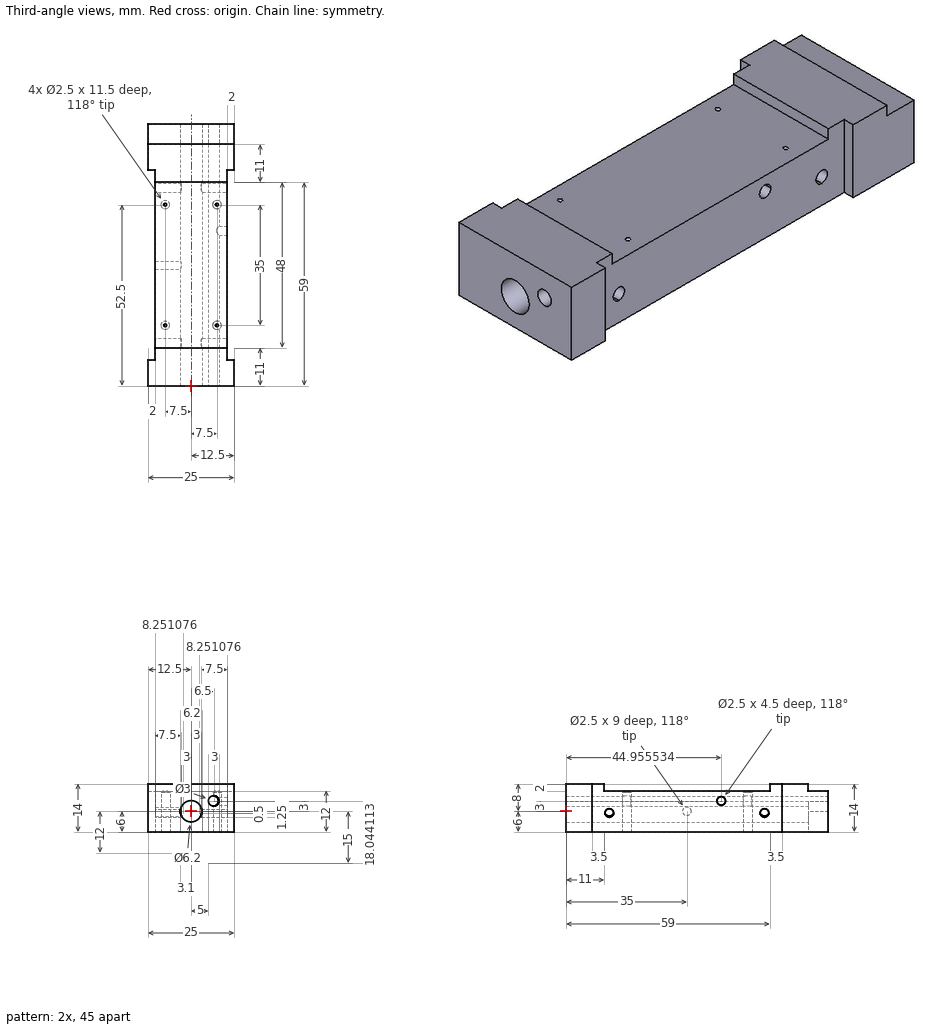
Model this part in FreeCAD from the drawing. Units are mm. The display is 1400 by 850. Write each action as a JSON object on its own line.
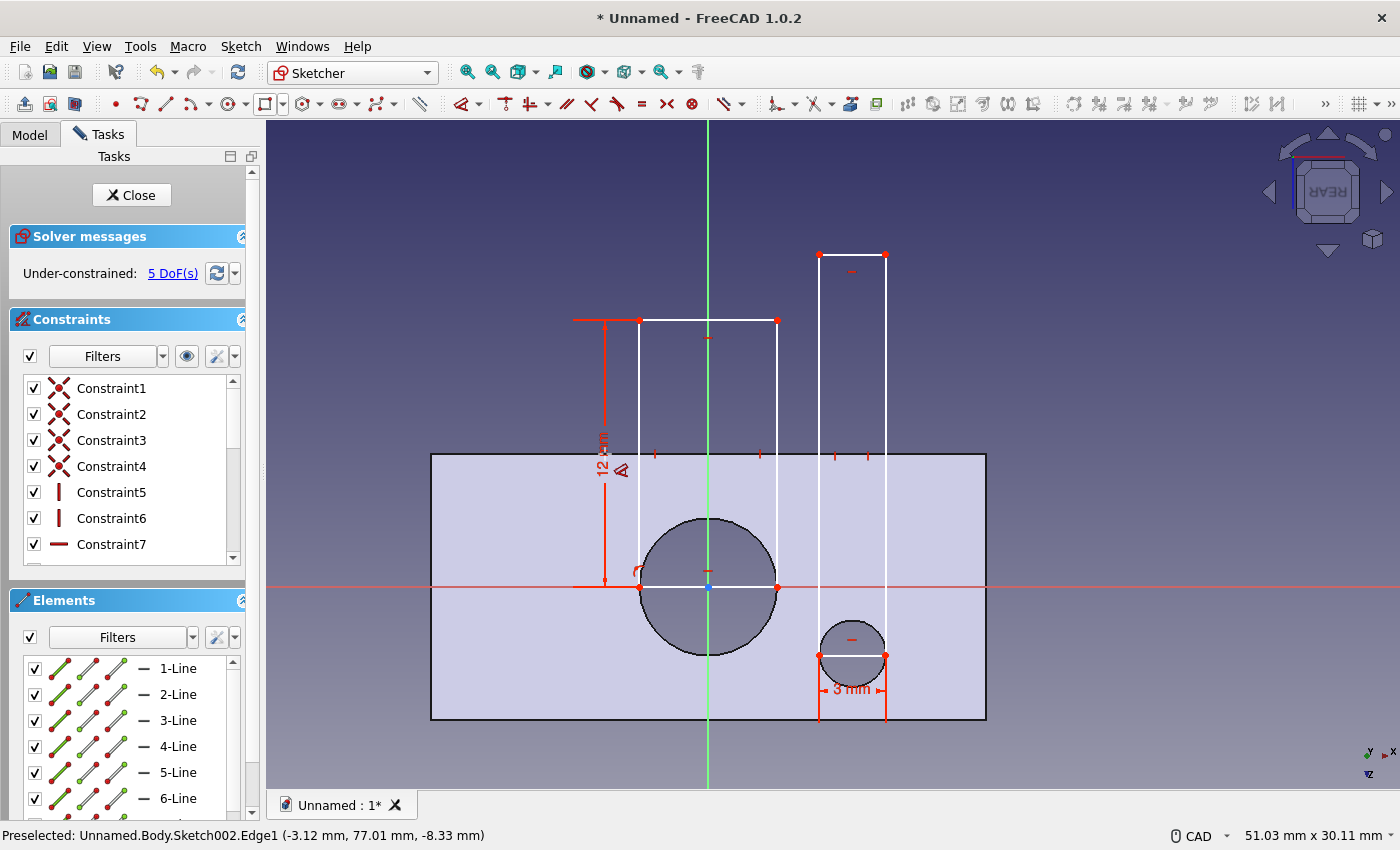
{"action": "left_click", "coordinate": [819, 255]}
{"action": "left_click", "coordinate": [764, 221]}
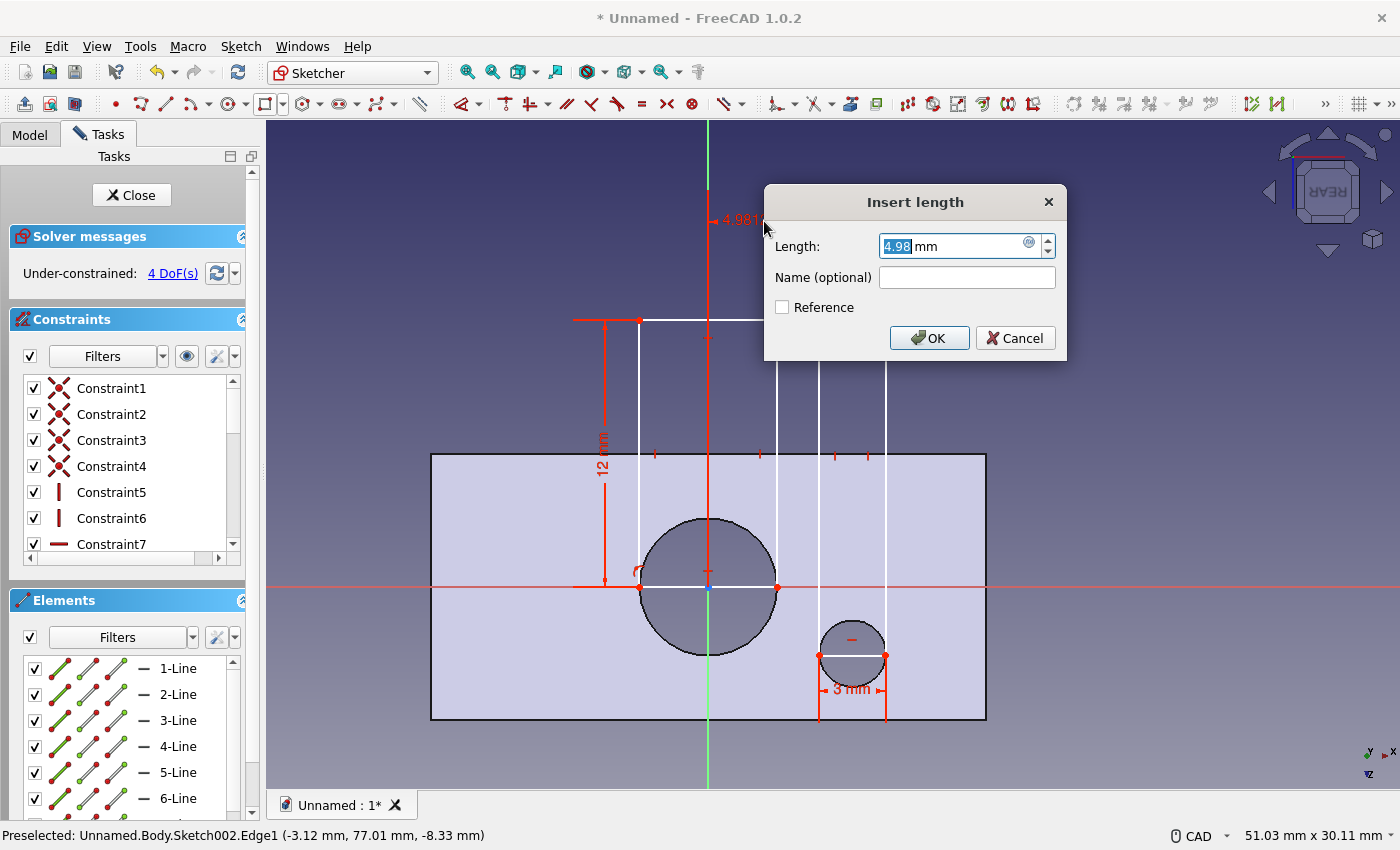
{"action": "type", "text": "5"}
{"action": "key", "text": "Return"}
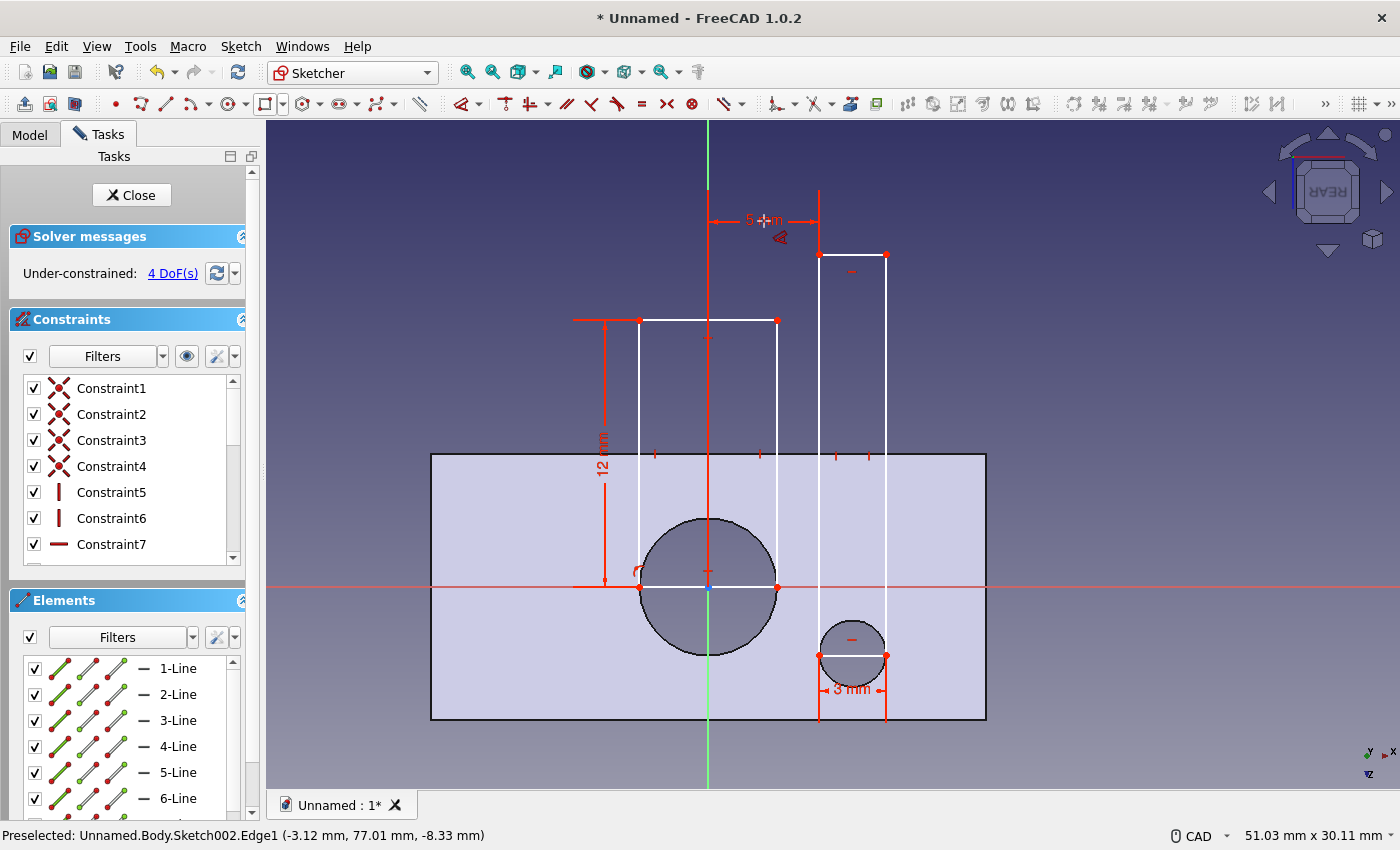
{"action": "left_click", "coordinate": [680, 587]}
{"action": "left_click", "coordinate": [676, 621]}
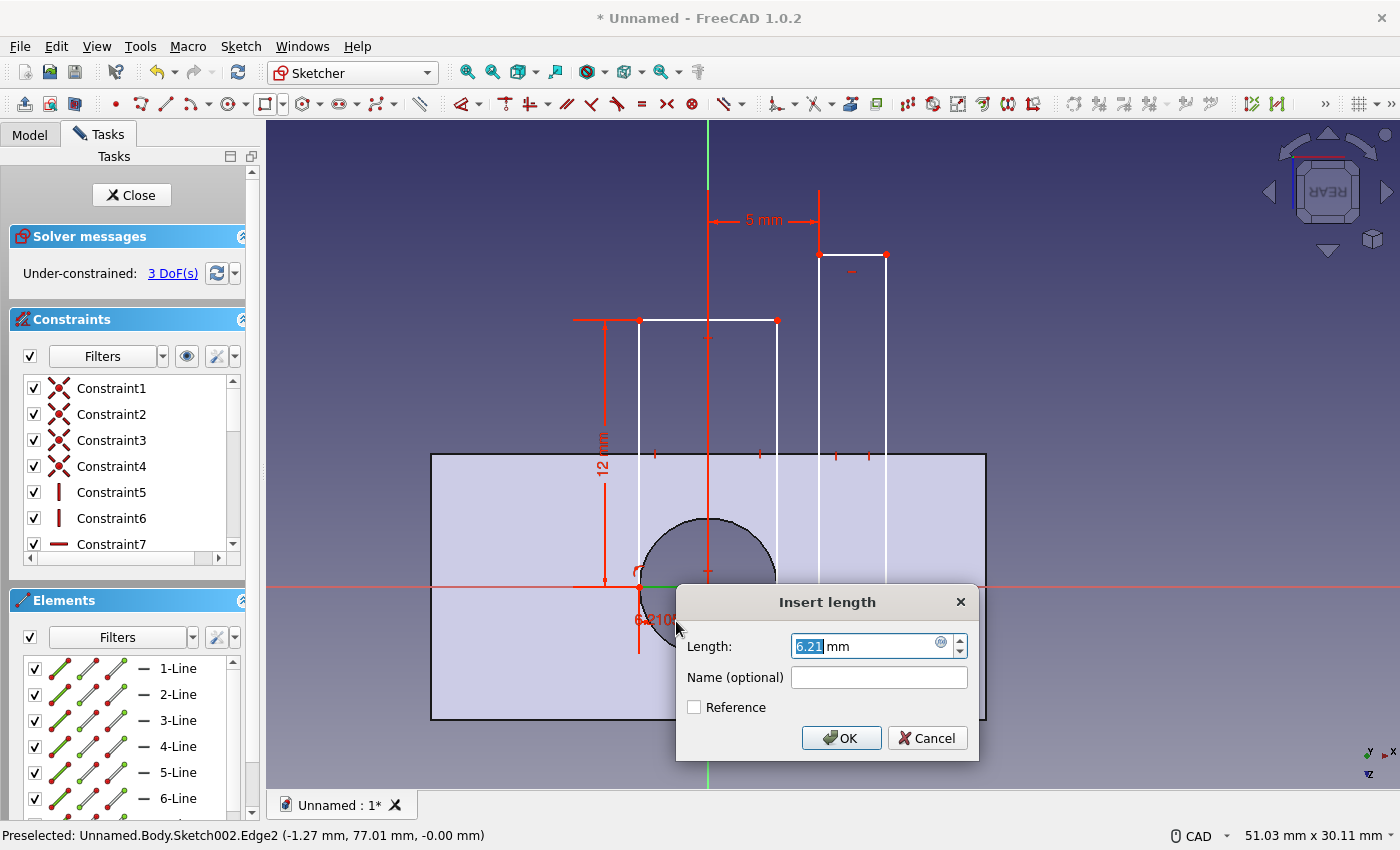
{"action": "type", "text": "6.2"}
{"action": "key", "text": "Return"}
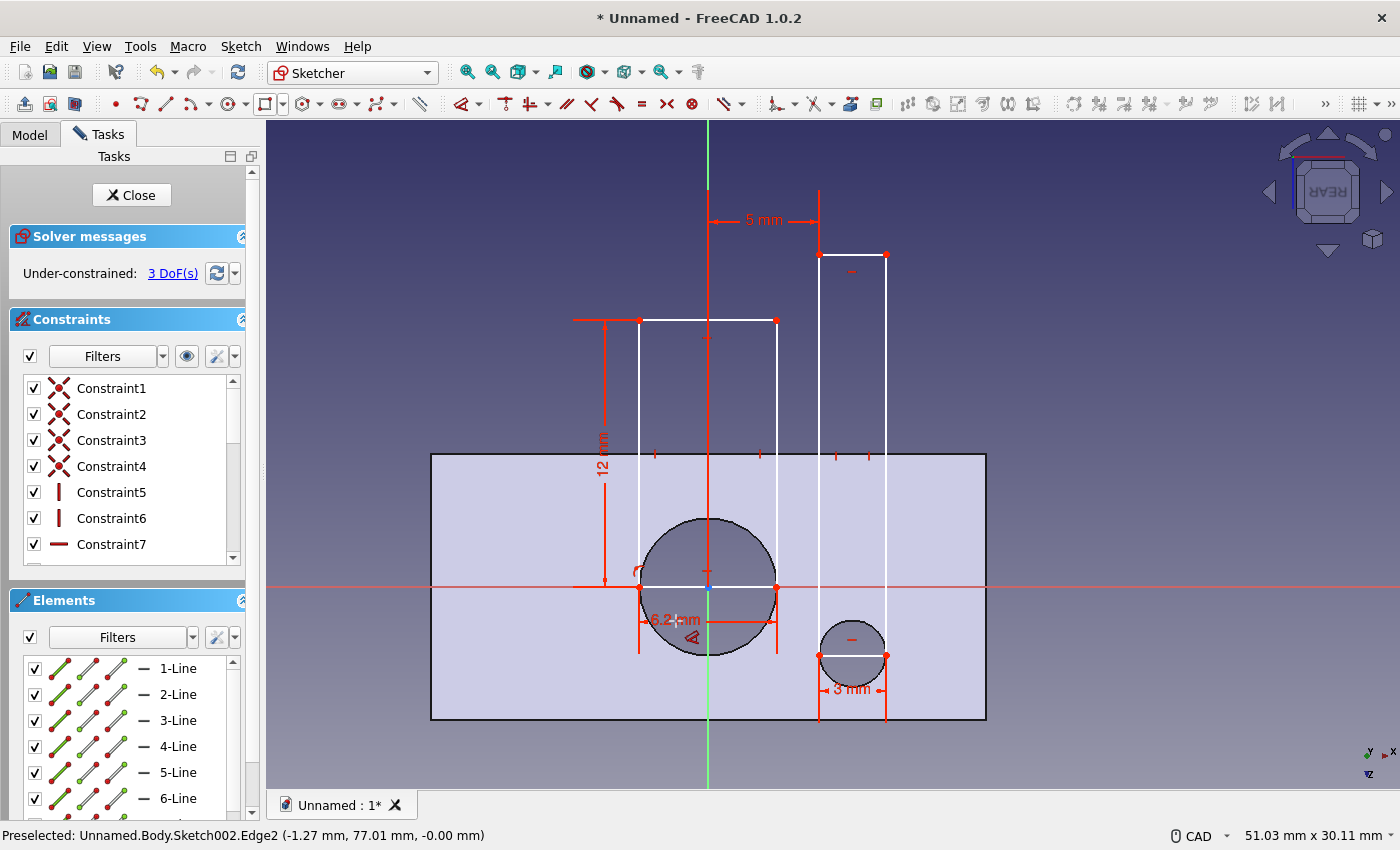
{"action": "left_click", "coordinate": [819, 255]}
{"action": "left_click", "coordinate": [853, 421]}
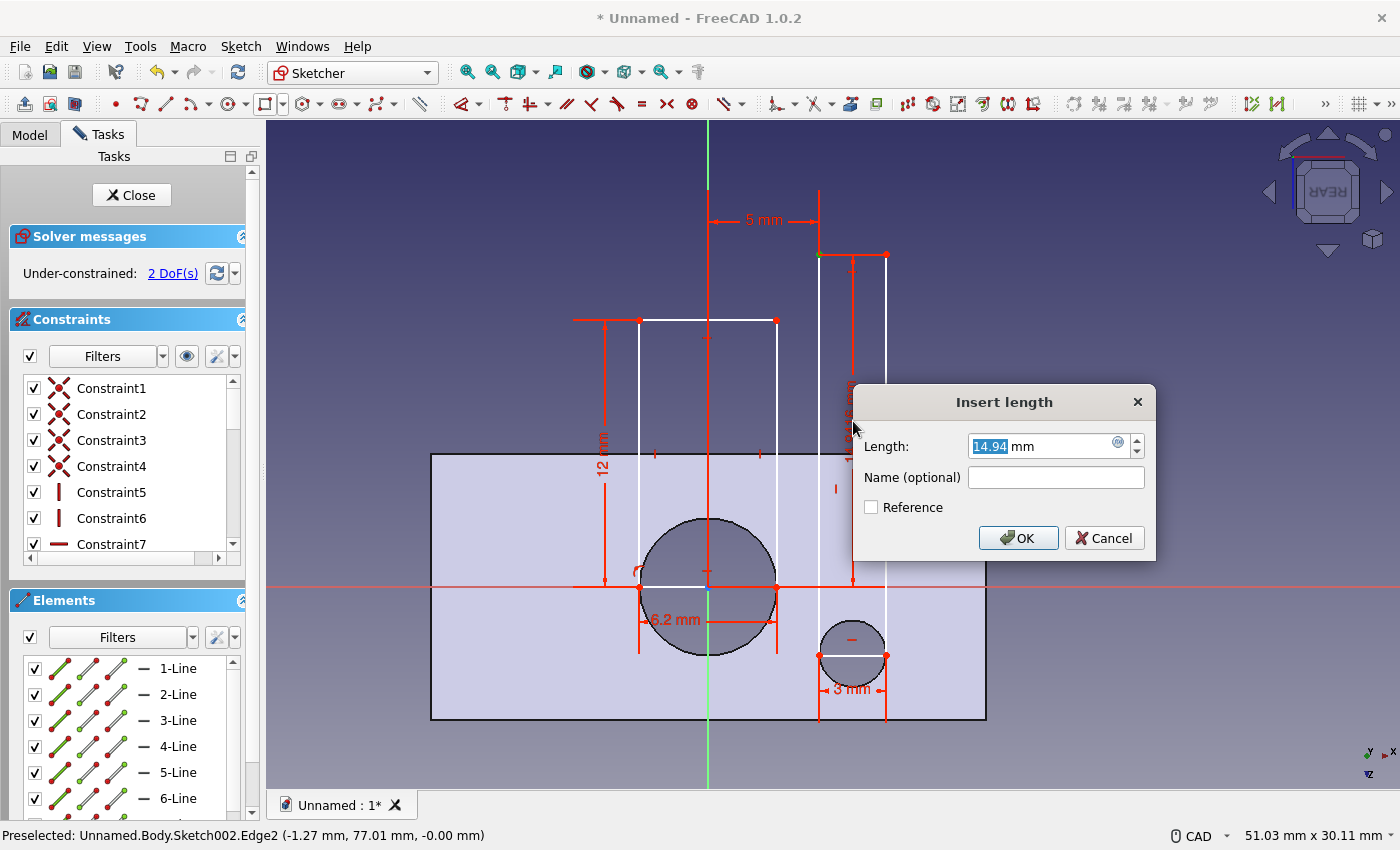
{"action": "type", "text": "15"}
{"action": "key", "text": "Return"}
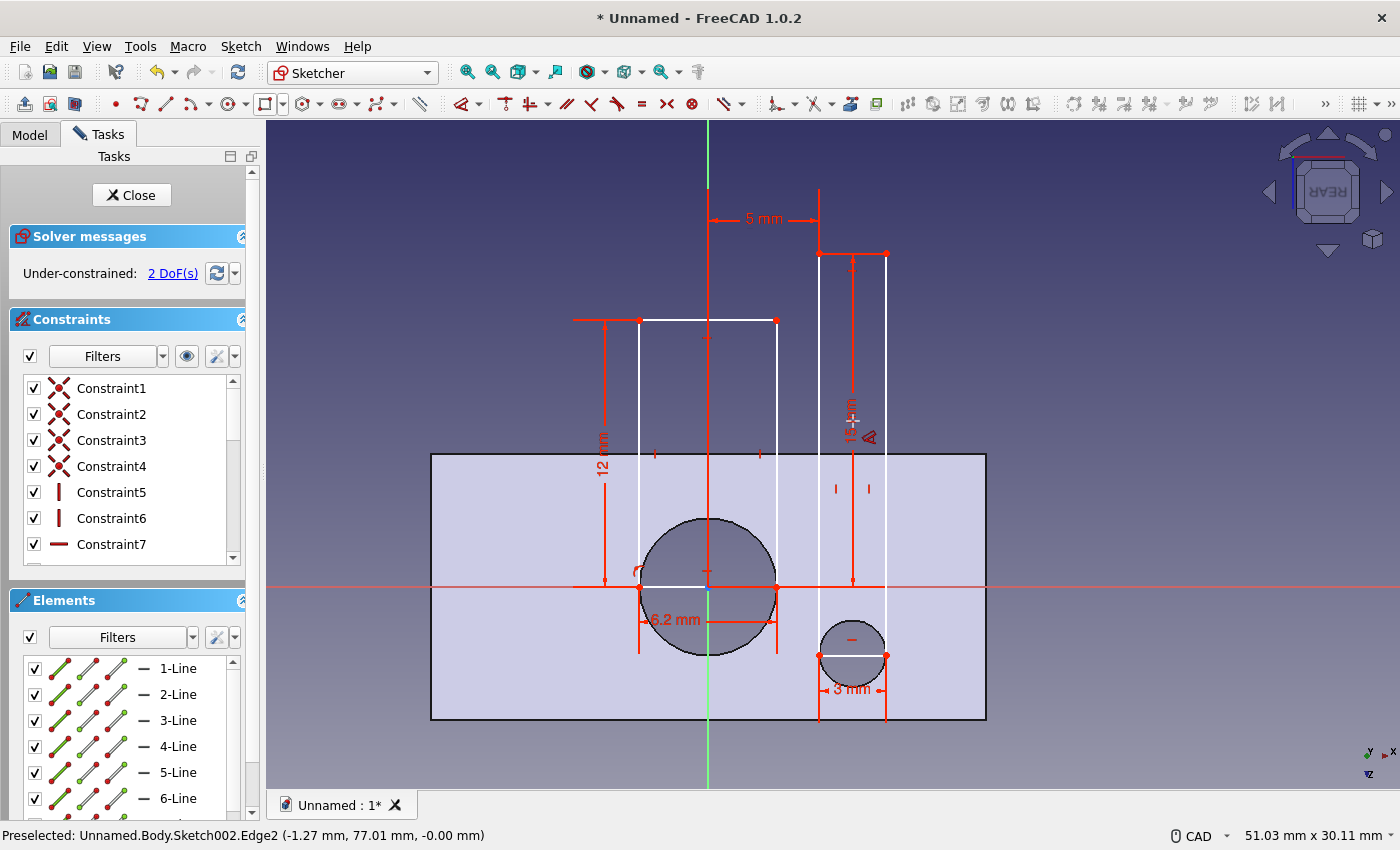
{"action": "left_click", "coordinate": [639, 320]}
{"action": "left_click", "coordinate": [674, 286]}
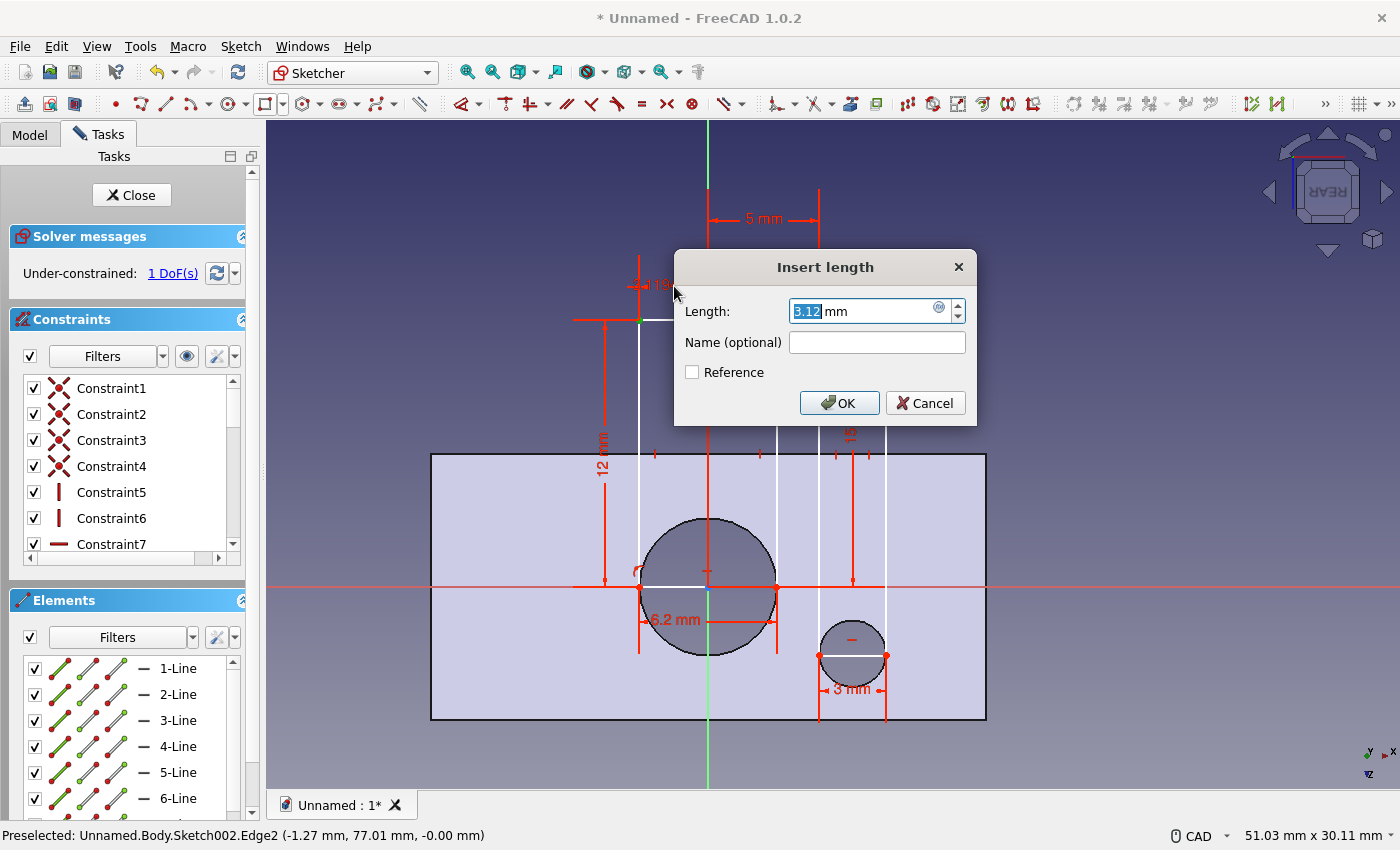
{"action": "type", "text": "3.1"}
{"action": "key", "text": "Return"}